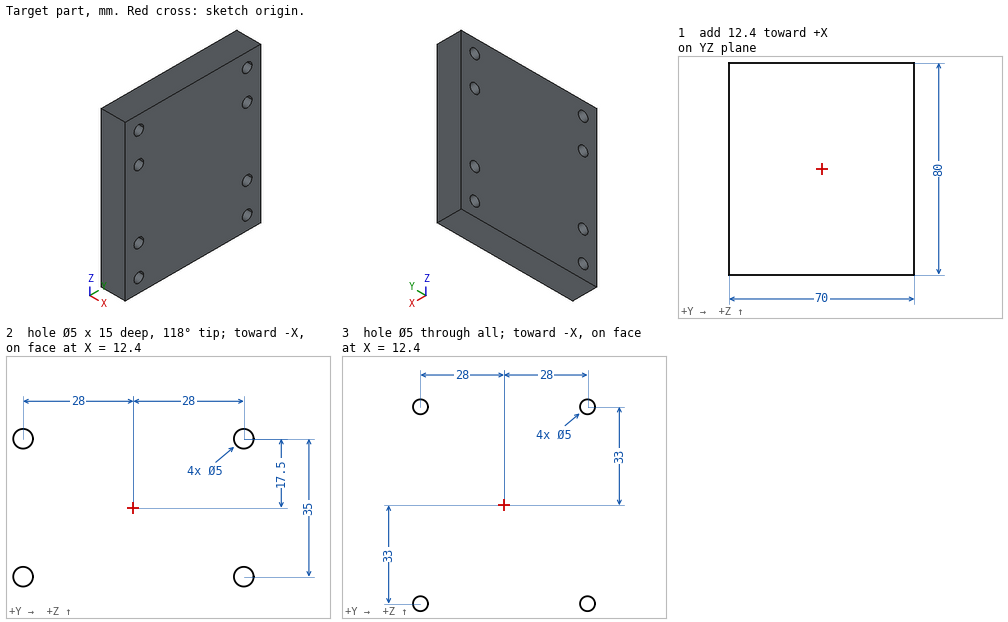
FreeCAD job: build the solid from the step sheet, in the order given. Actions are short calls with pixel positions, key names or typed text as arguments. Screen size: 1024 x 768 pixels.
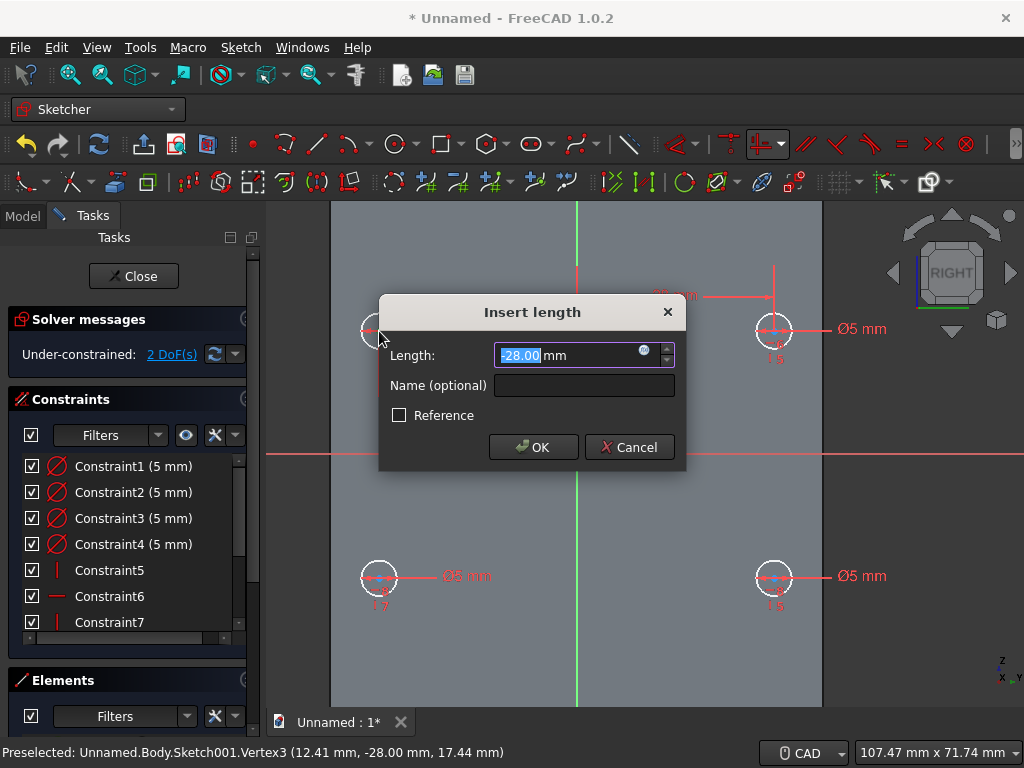
text(-28)
key(Return)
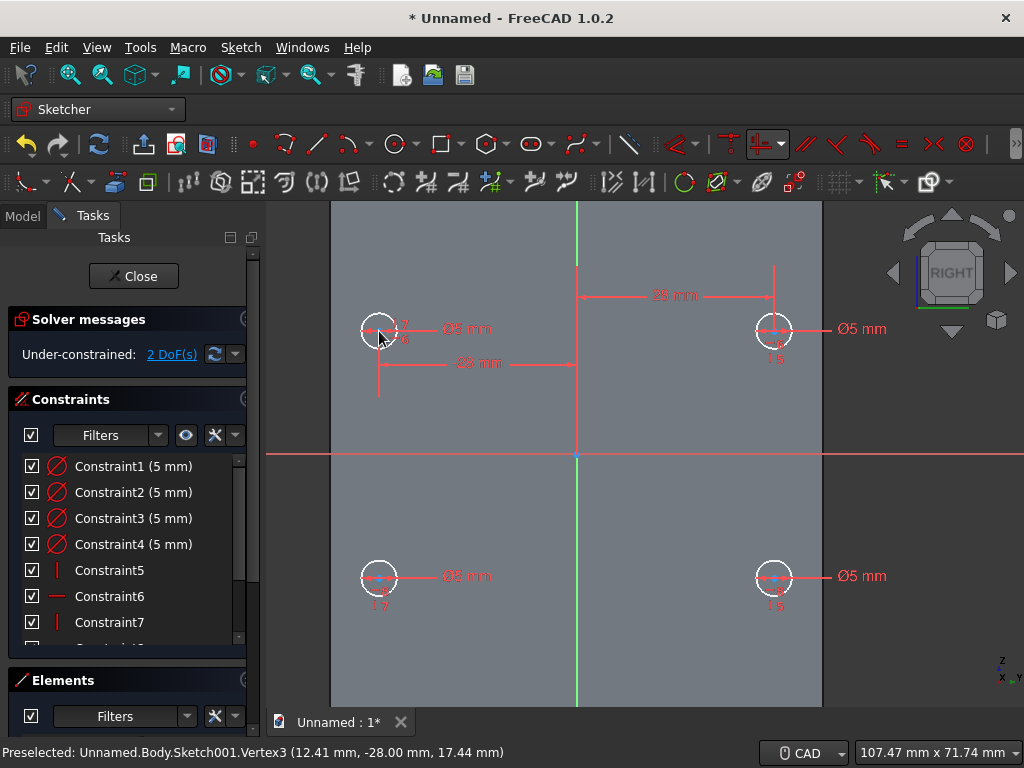
click(774, 331)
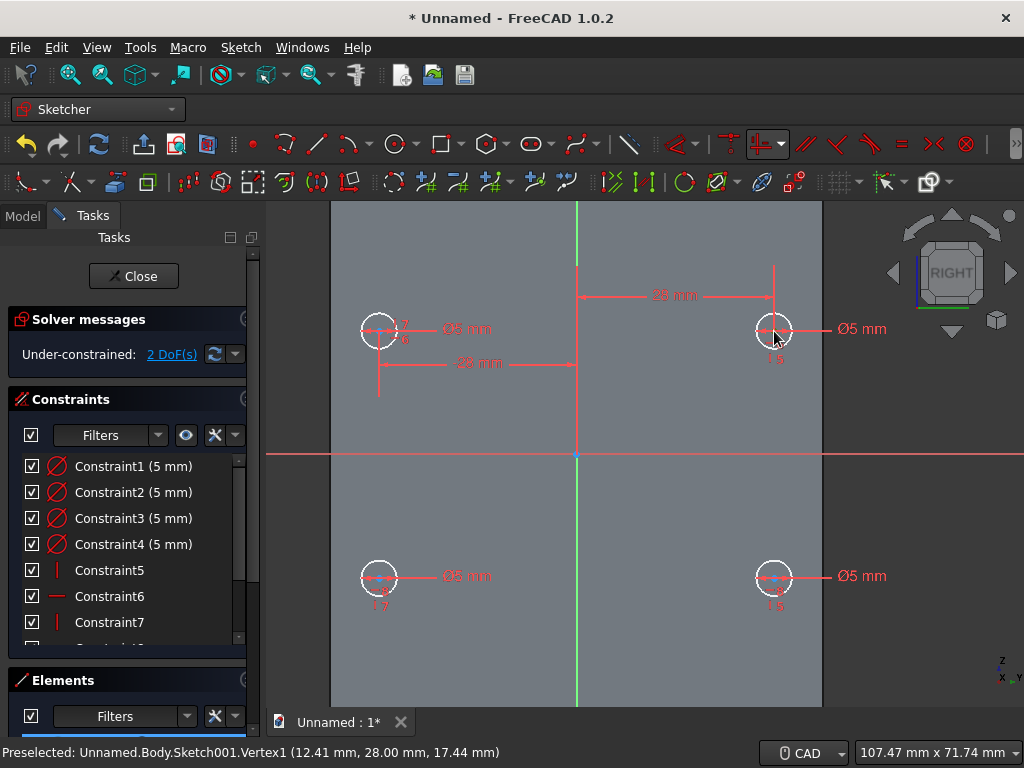
click(774, 578)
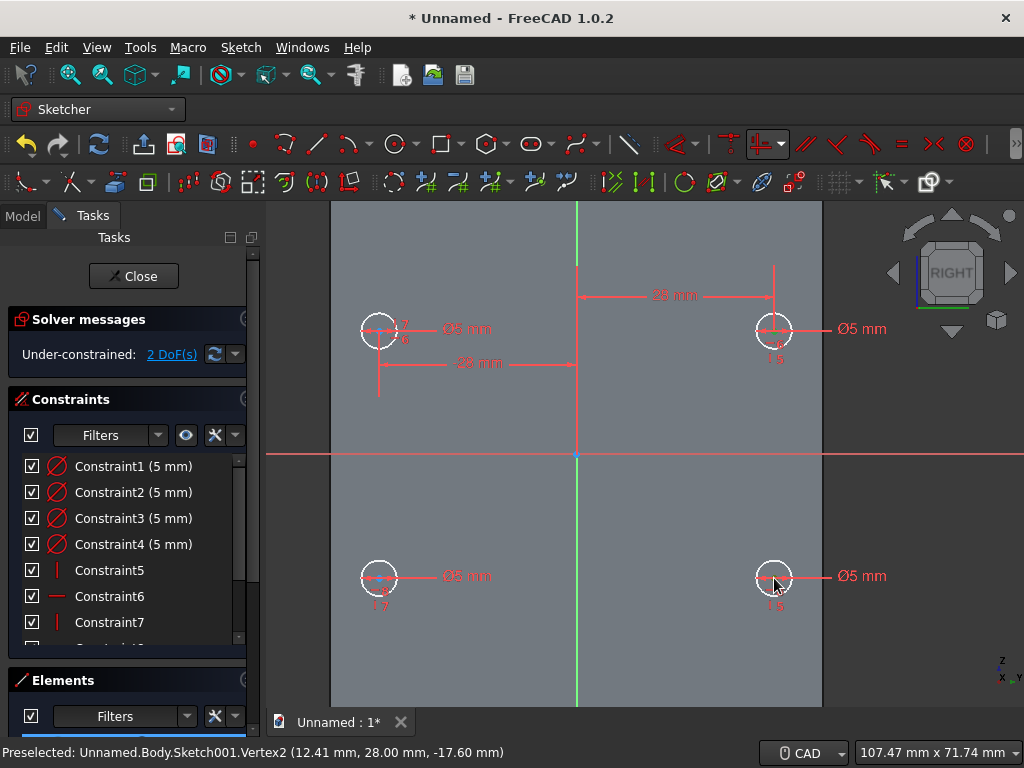
key(i)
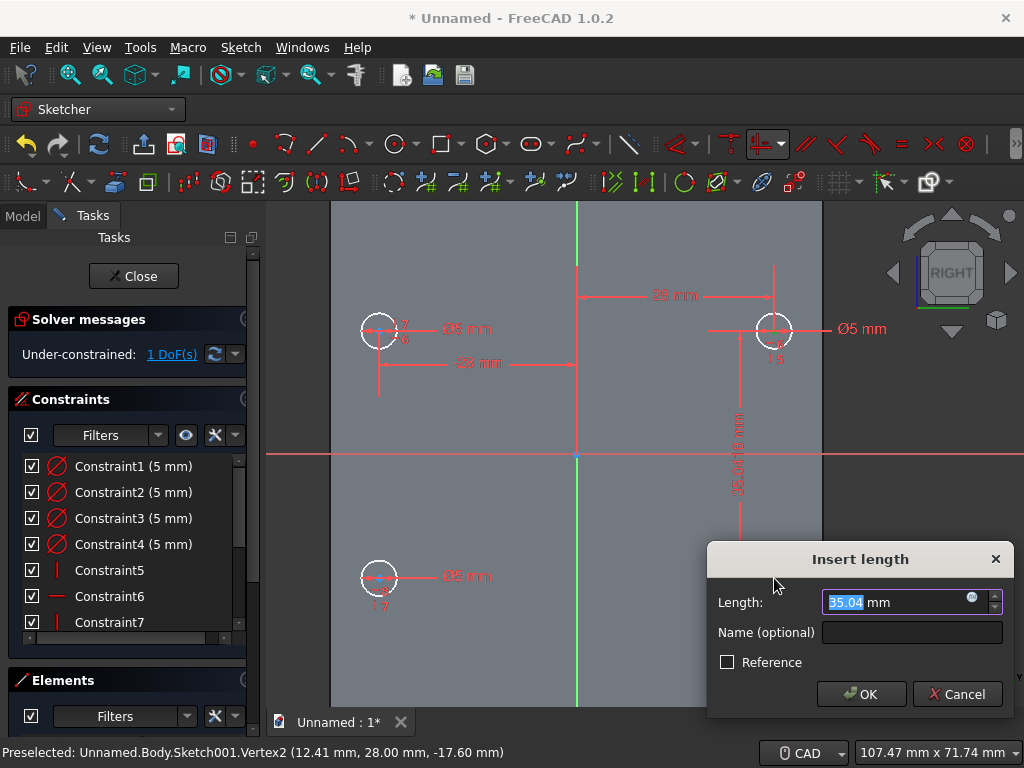
text(35)
key(Return)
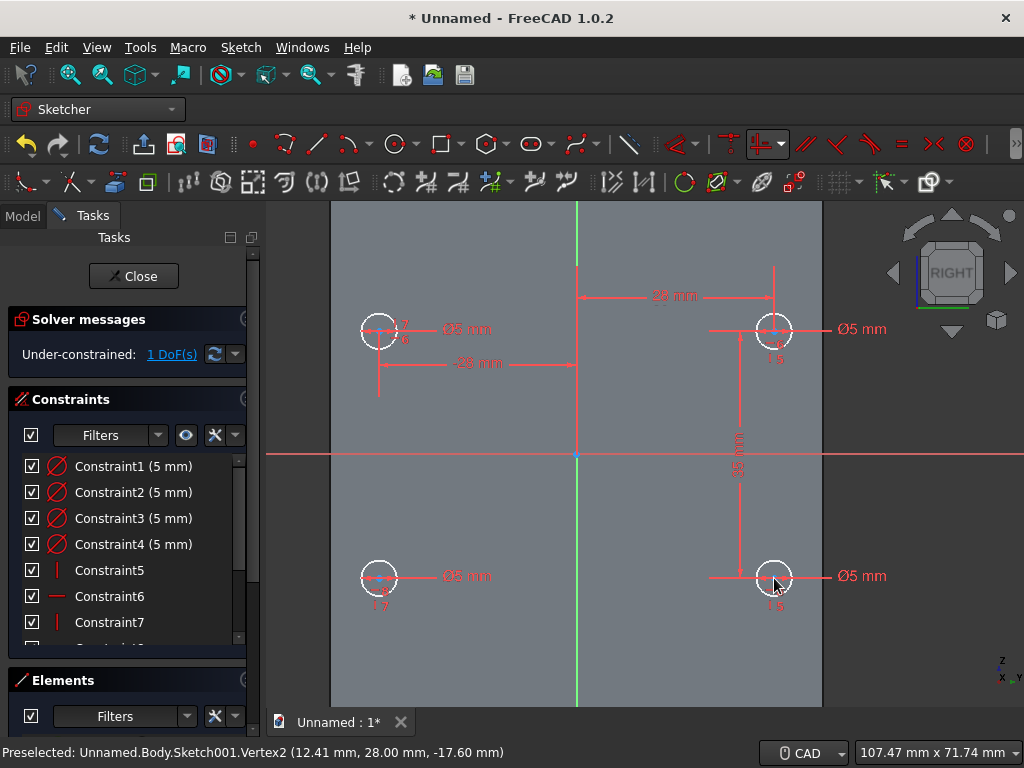
click(774, 331)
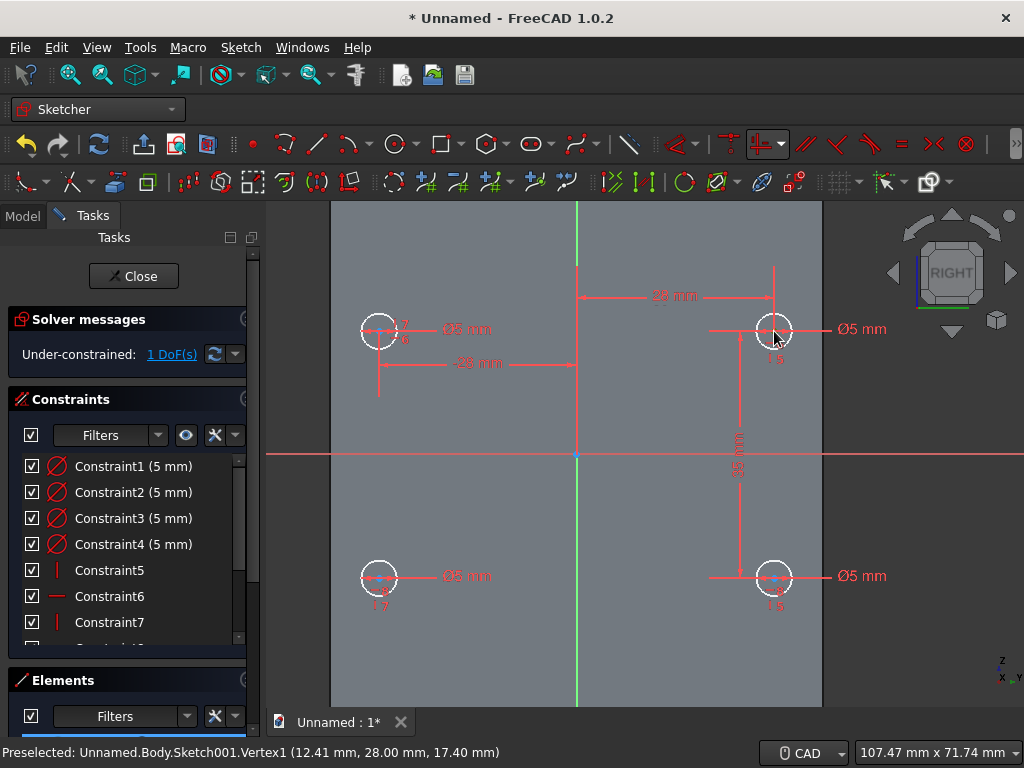
key(i)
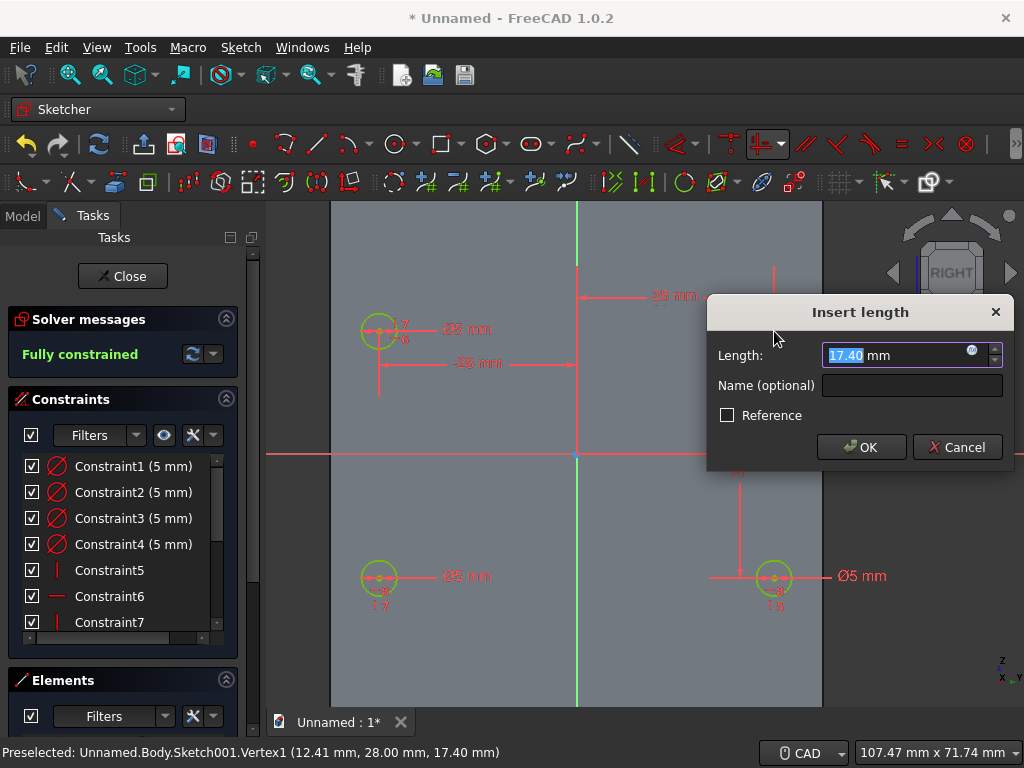
text(17.5)
key(Return)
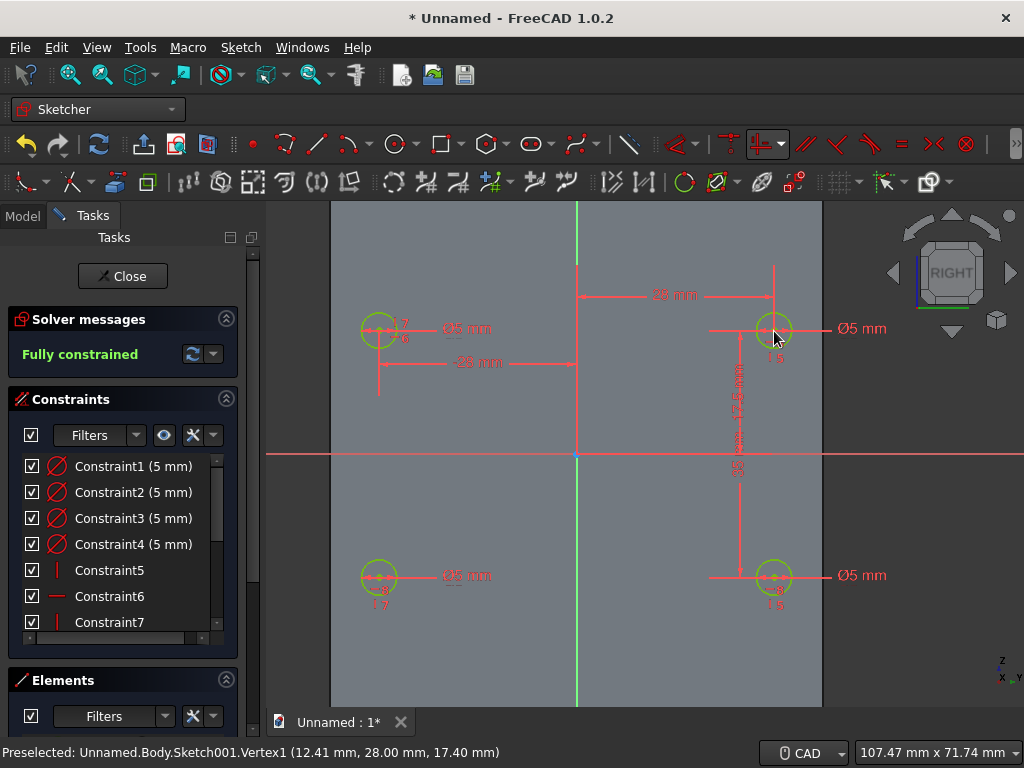
click(123, 276)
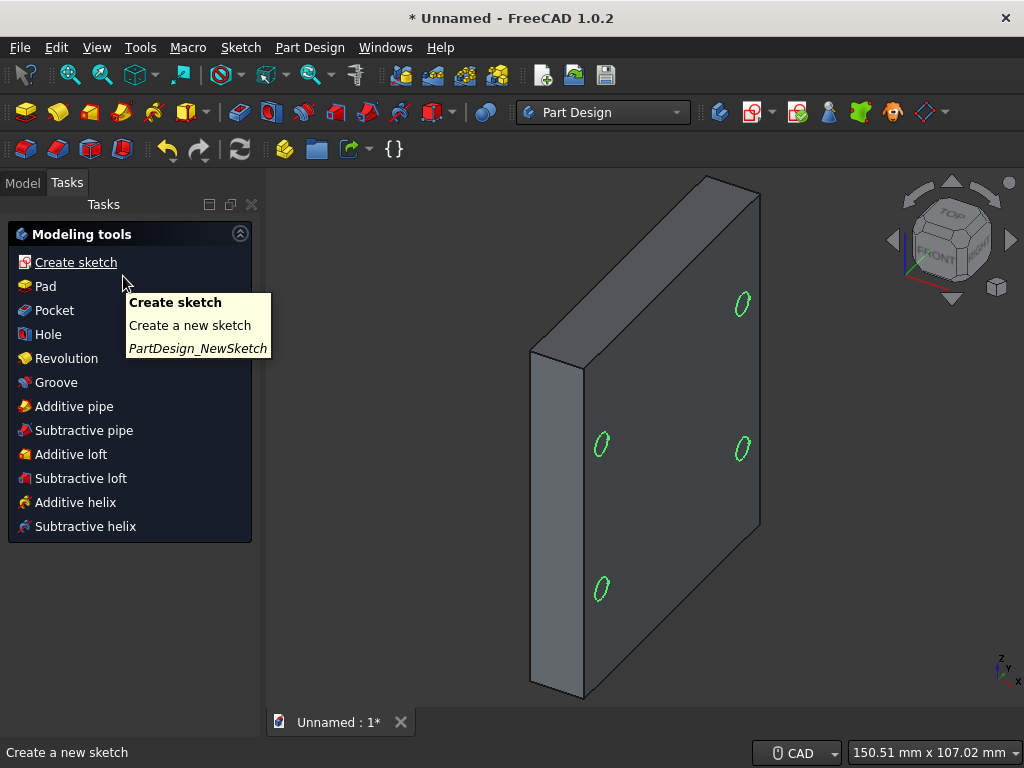
click(272, 112)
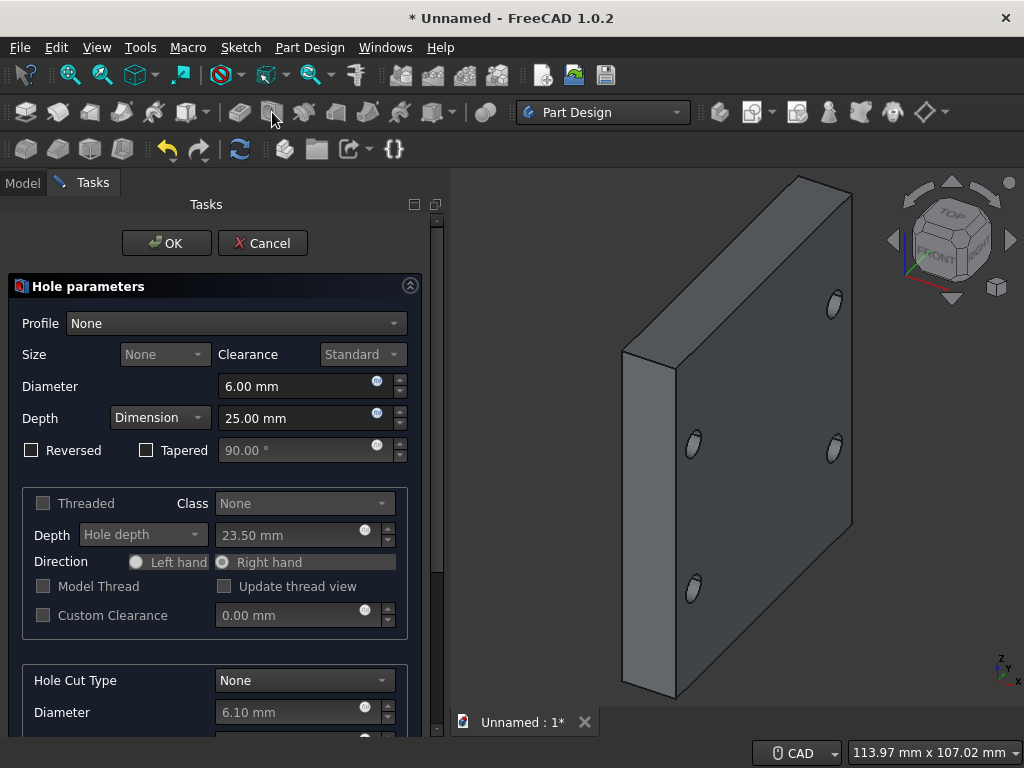
triple_click(305, 386)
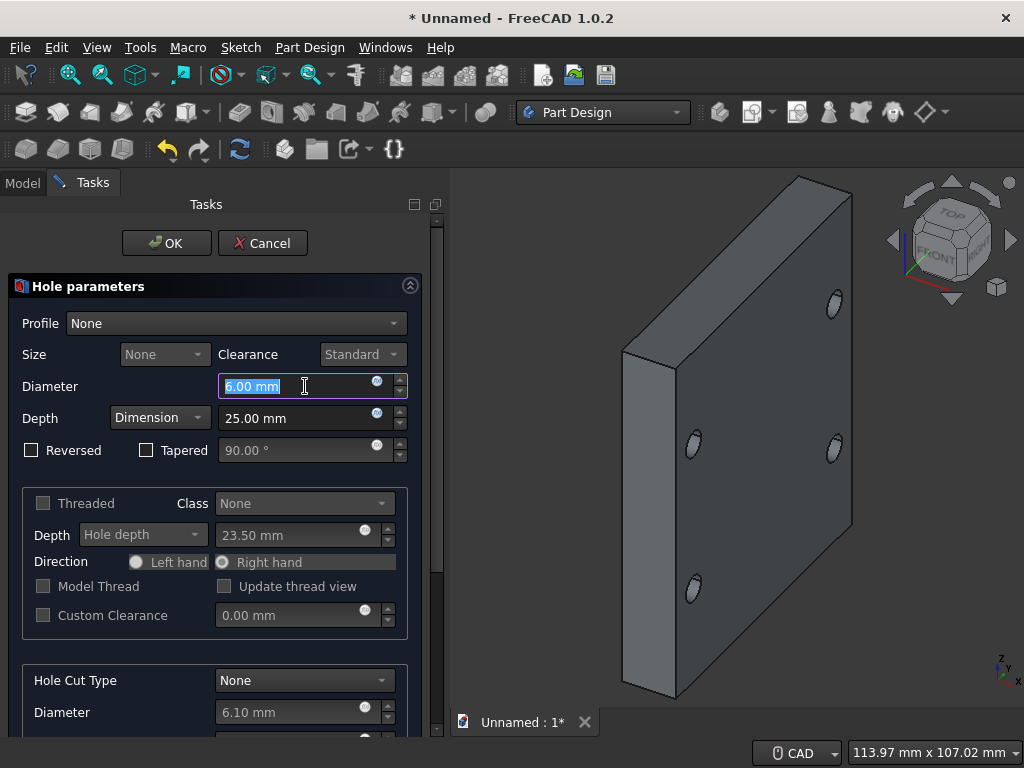
text(5)
key(Tab)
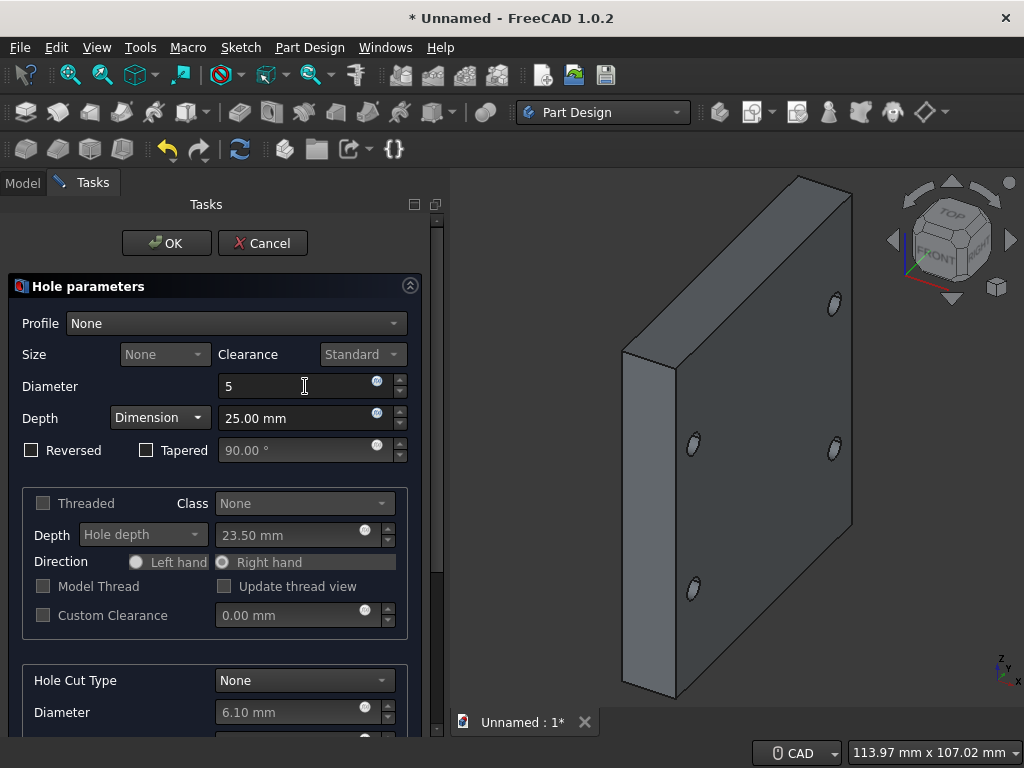
triple_click(305, 418)